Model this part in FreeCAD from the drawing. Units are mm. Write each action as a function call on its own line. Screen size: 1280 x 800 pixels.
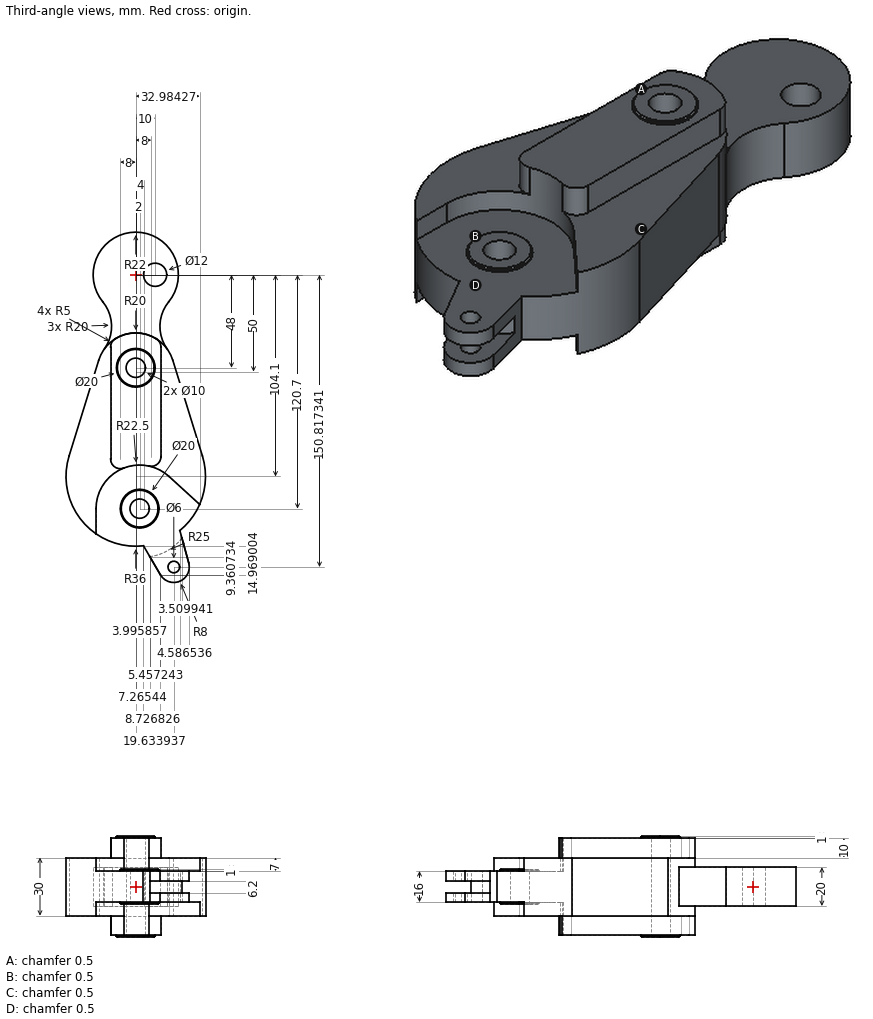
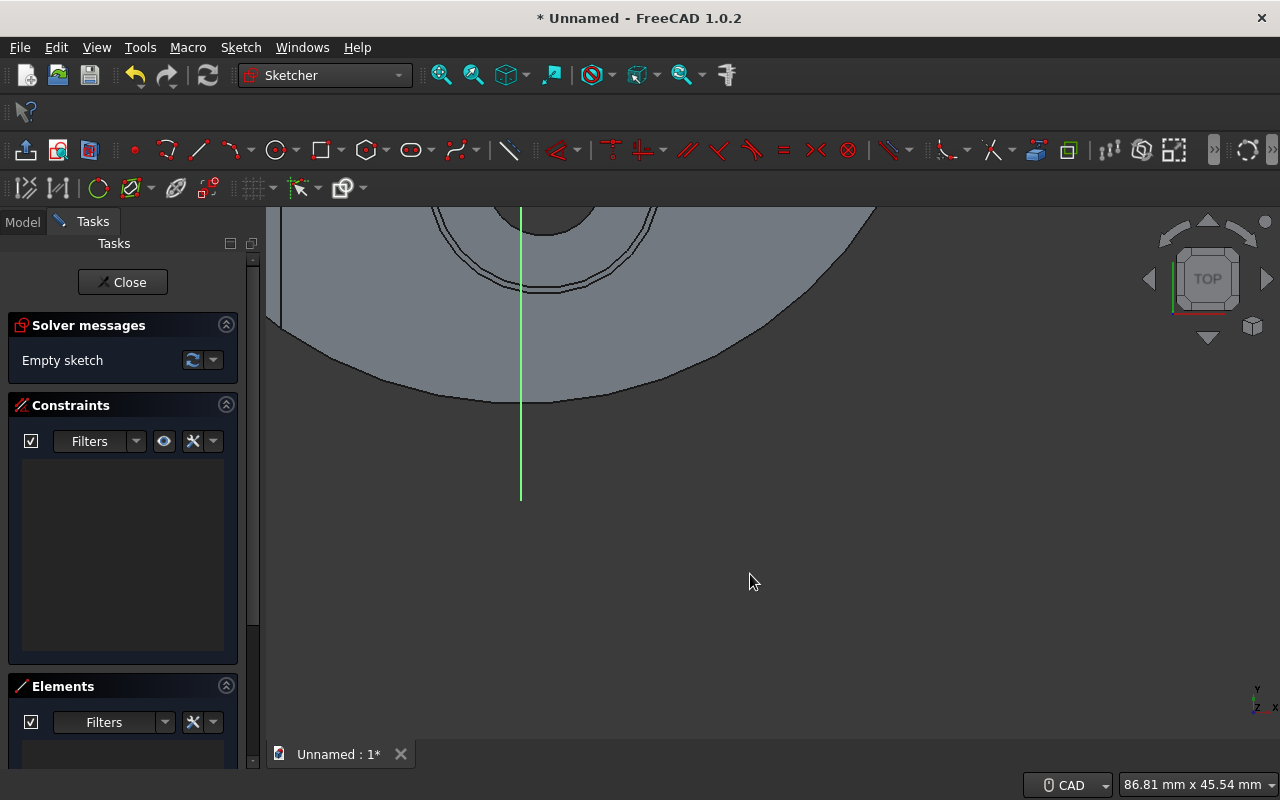
click(200, 150)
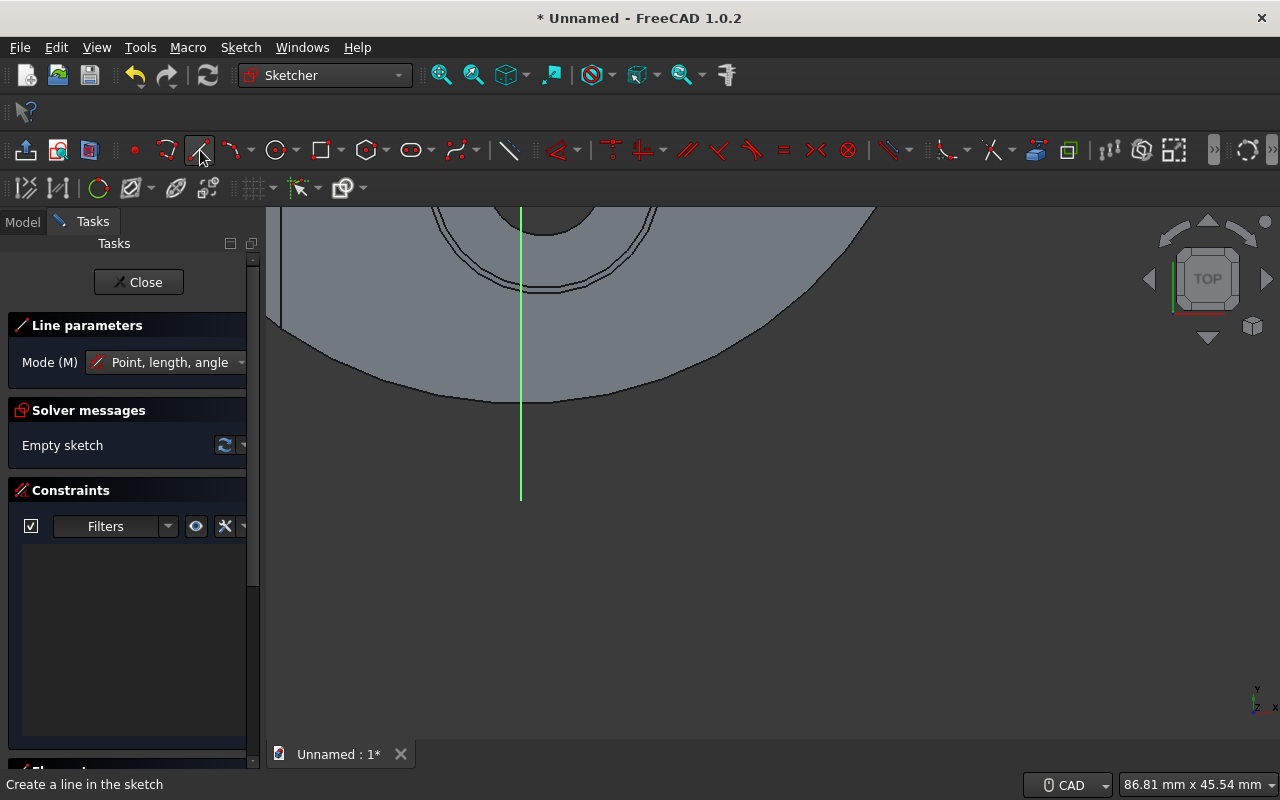
click(568, 401)
click(670, 576)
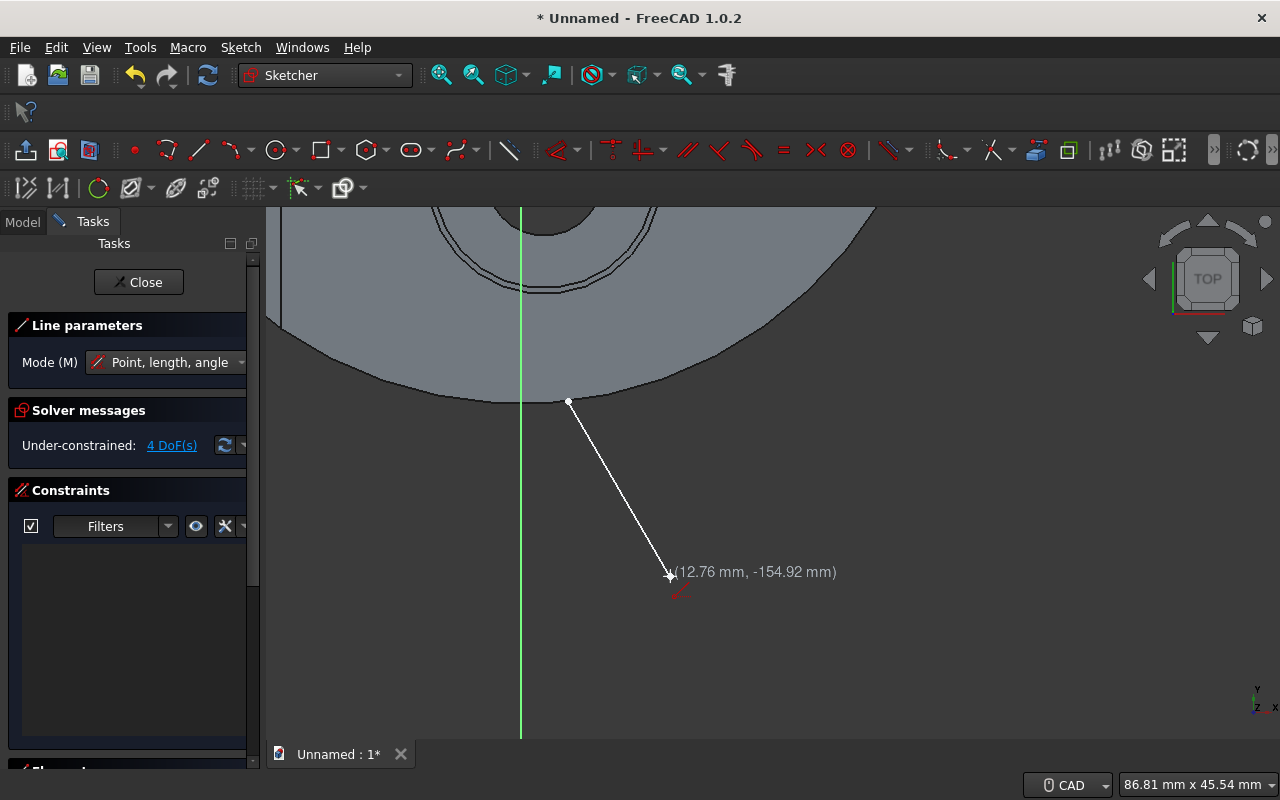
click(840, 504)
click(787, 309)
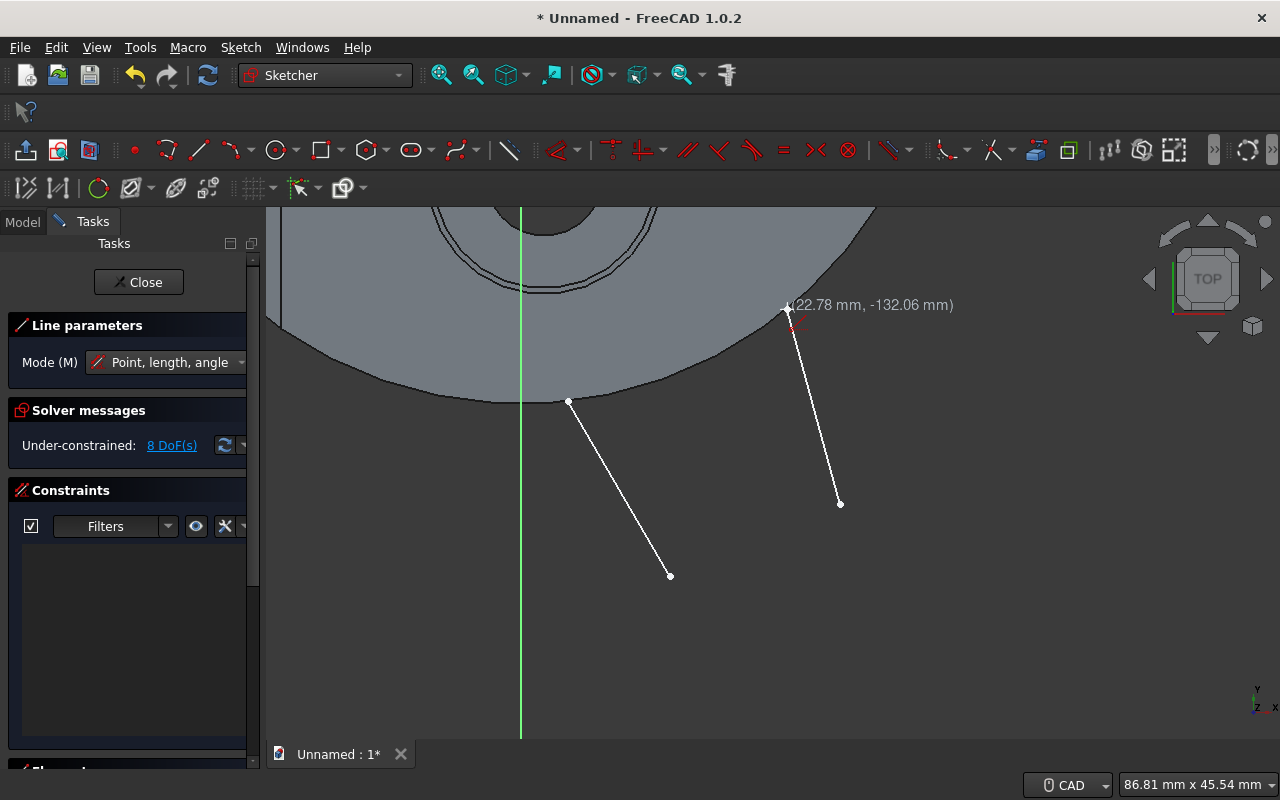
click(232, 150)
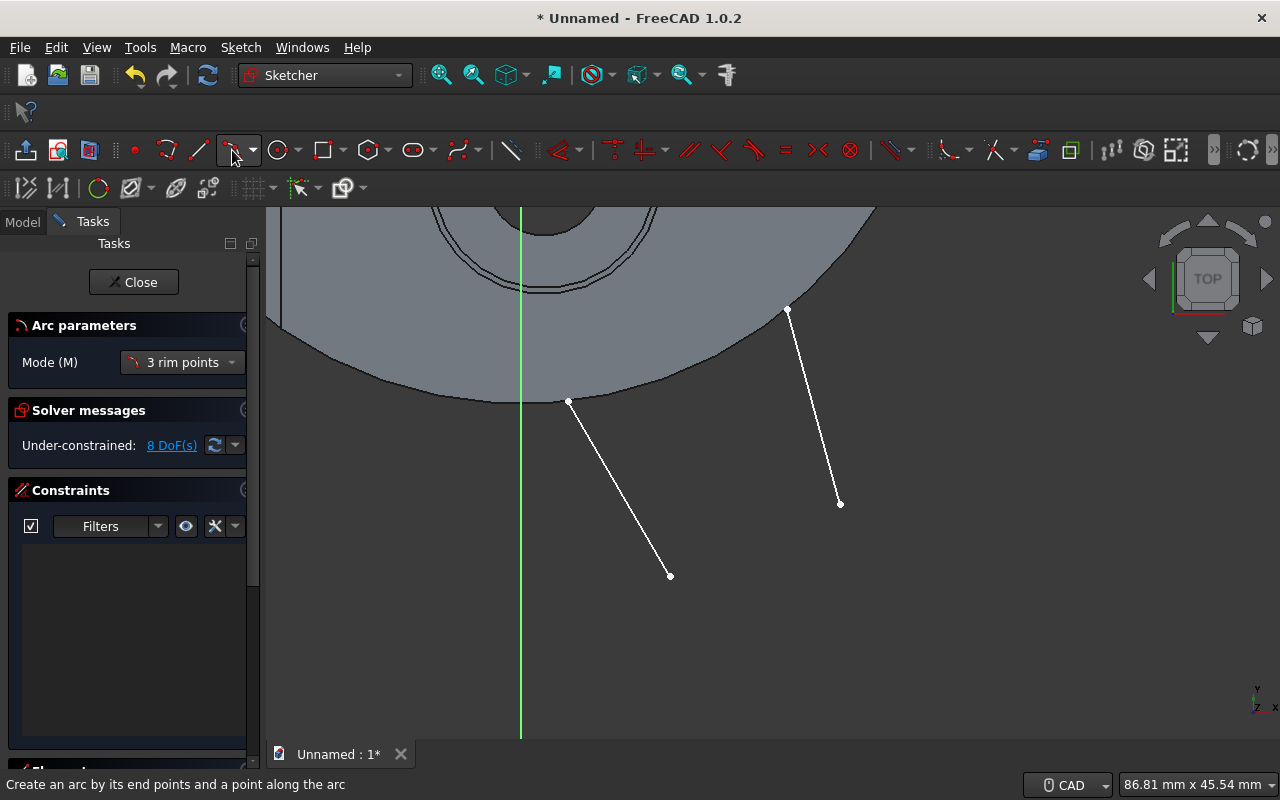
click(670, 577)
click(840, 505)
click(787, 615)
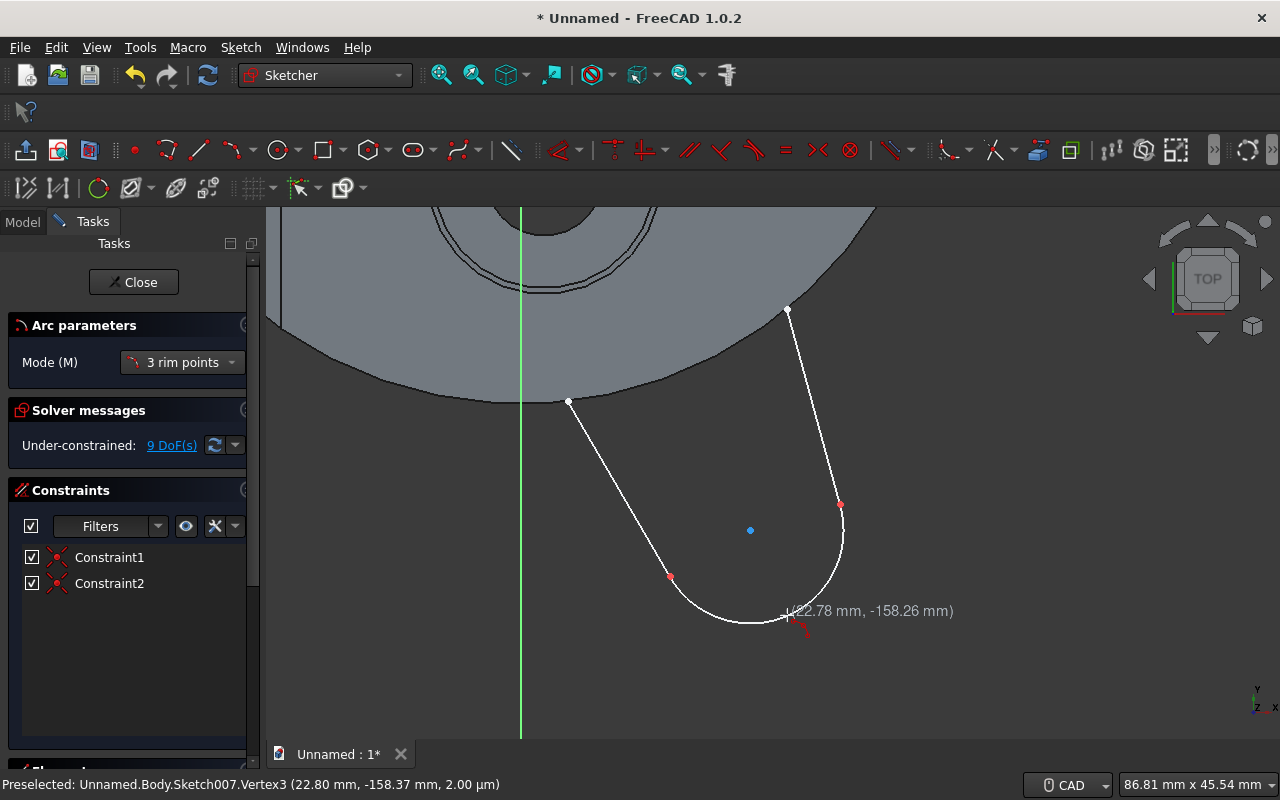
click(787, 310)
click(568, 402)
click(684, 371)
key(Escape)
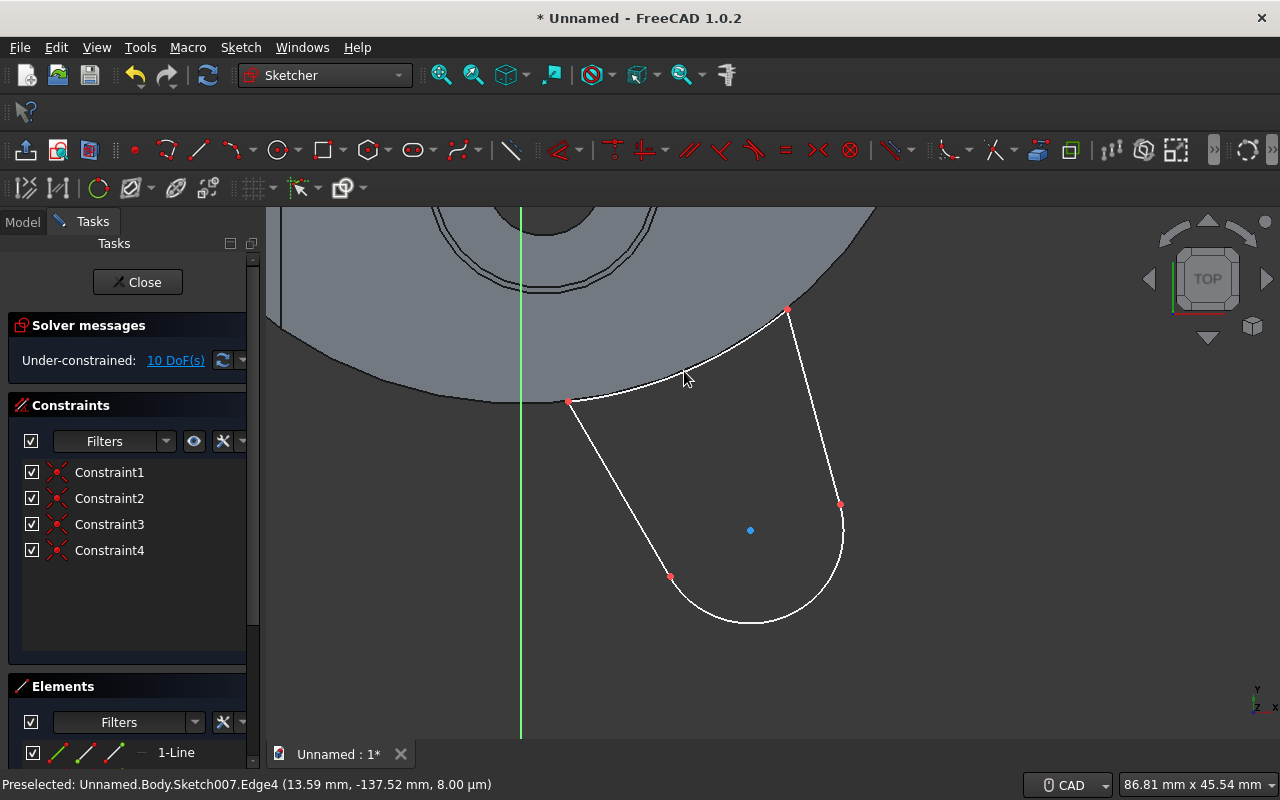
click(599, 454)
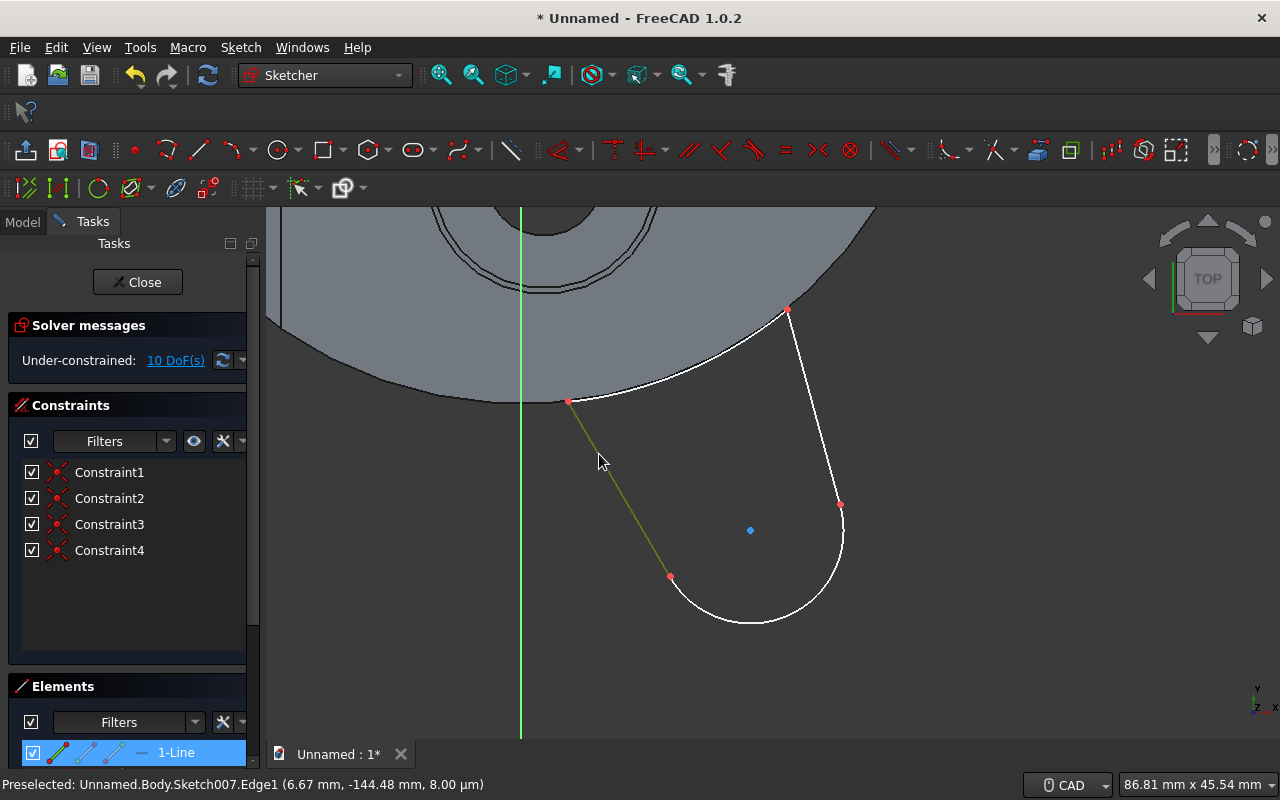
click(734, 622)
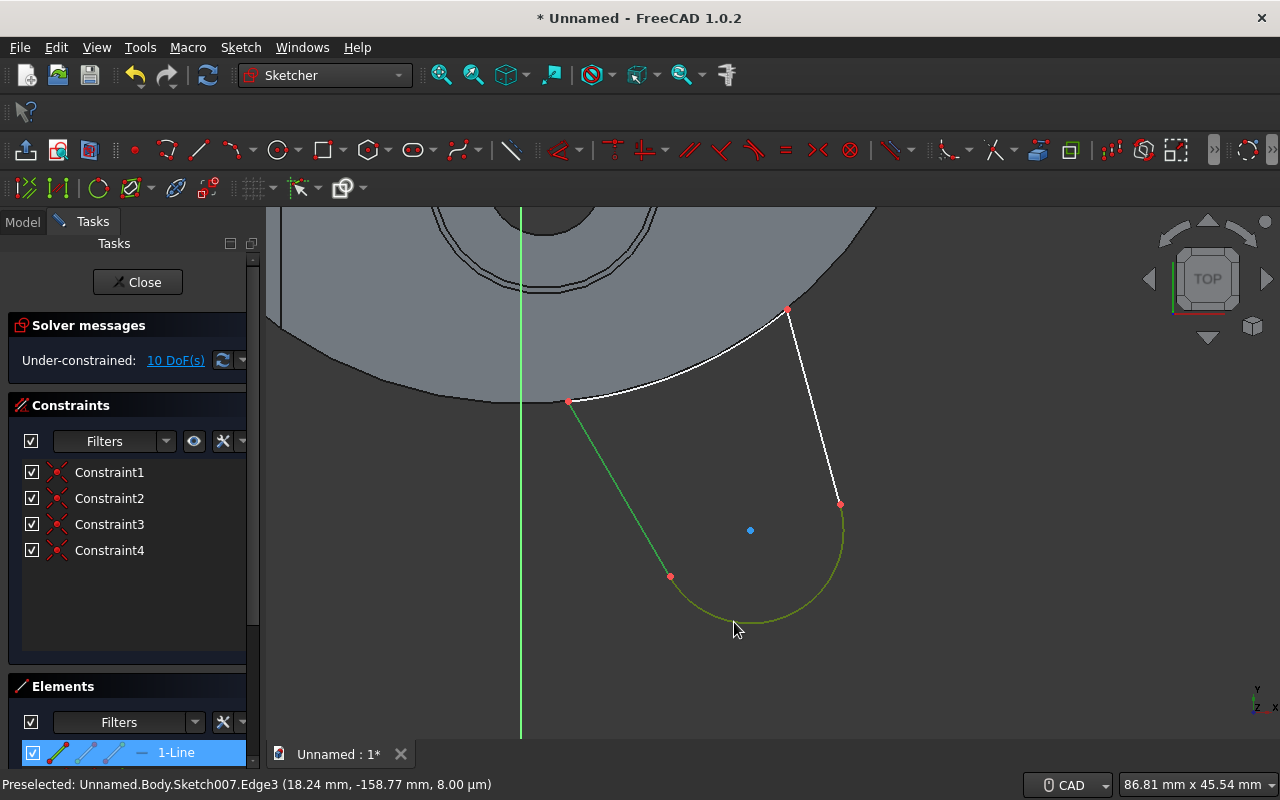
click(754, 150)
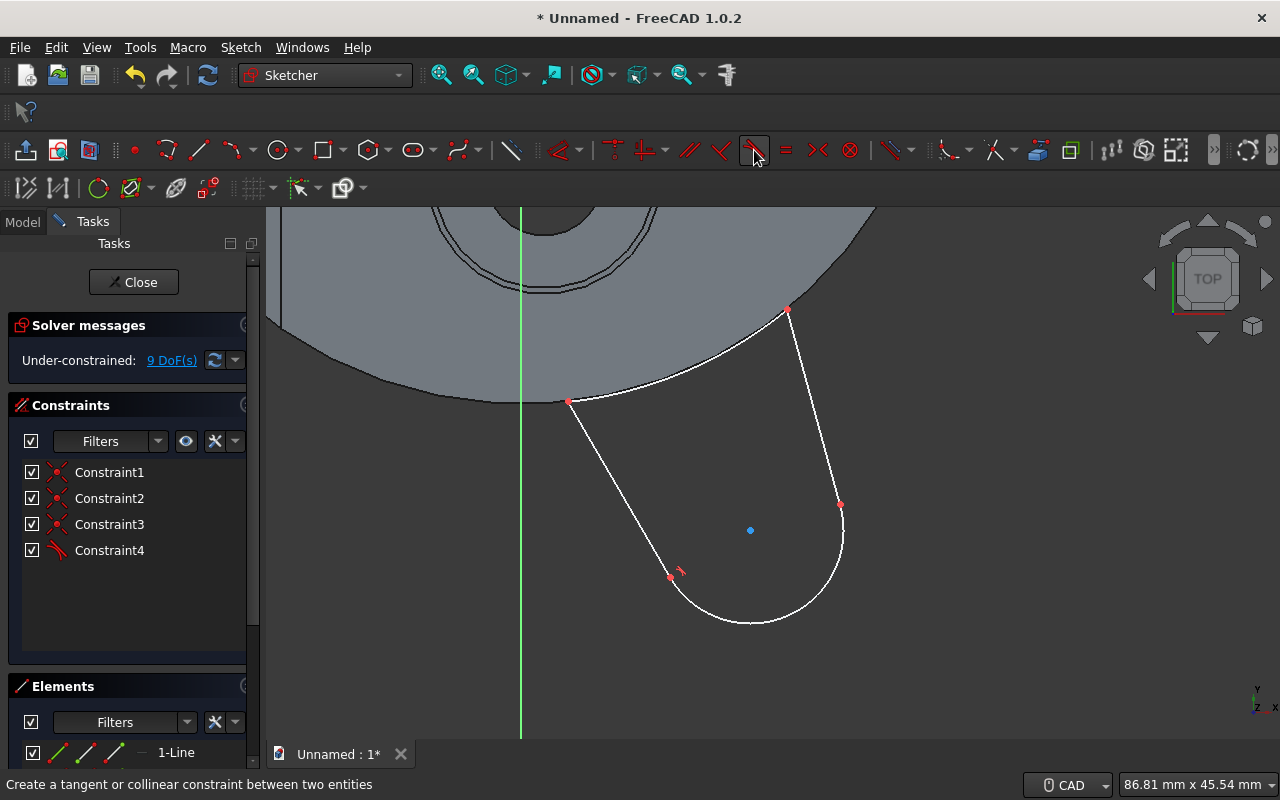
click(824, 446)